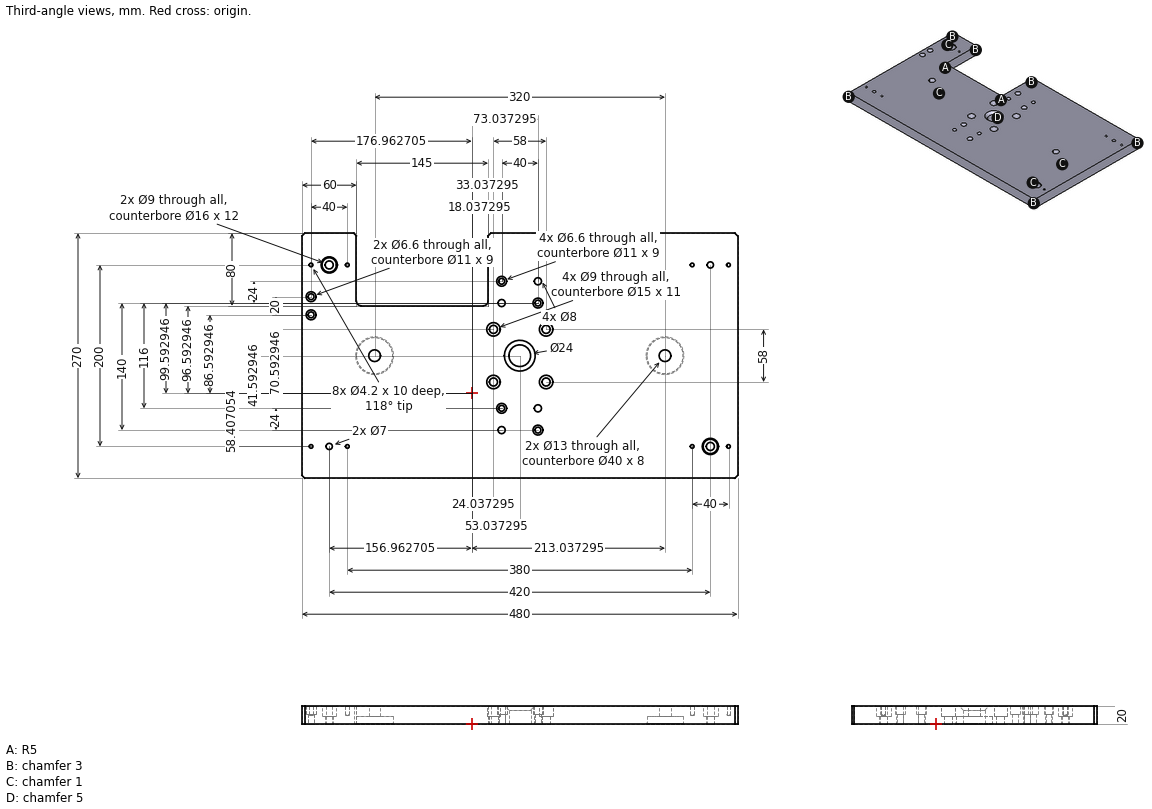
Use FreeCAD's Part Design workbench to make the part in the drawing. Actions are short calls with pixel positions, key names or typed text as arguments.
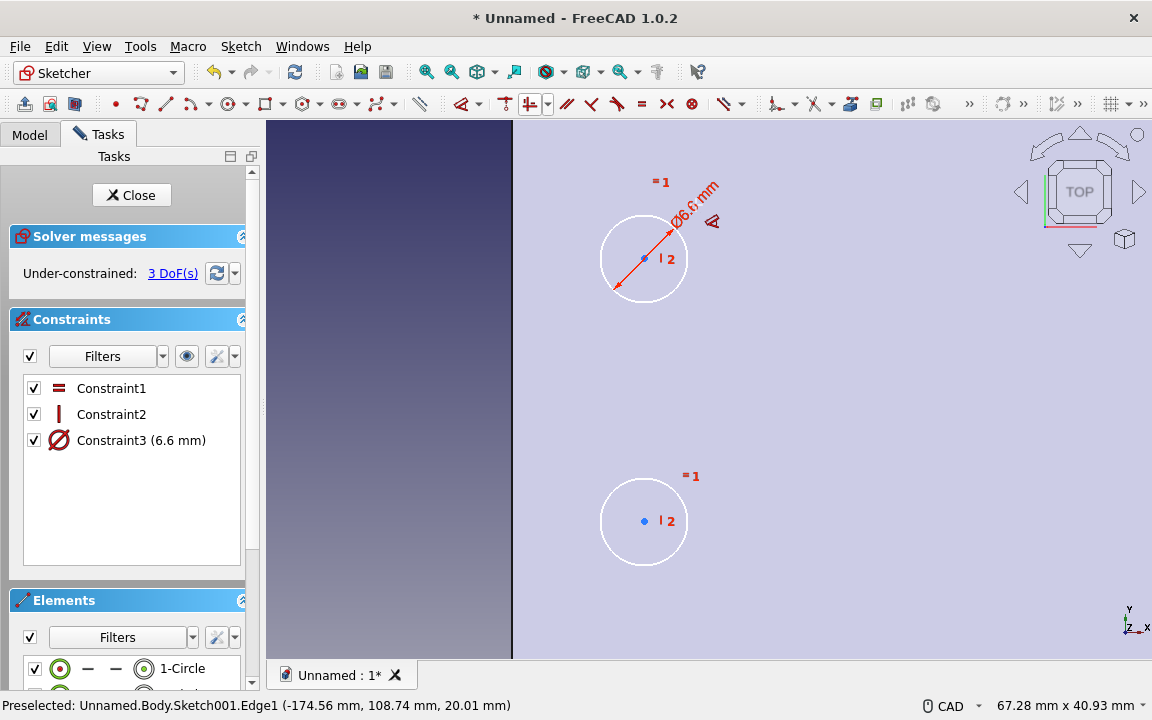
click(644, 259)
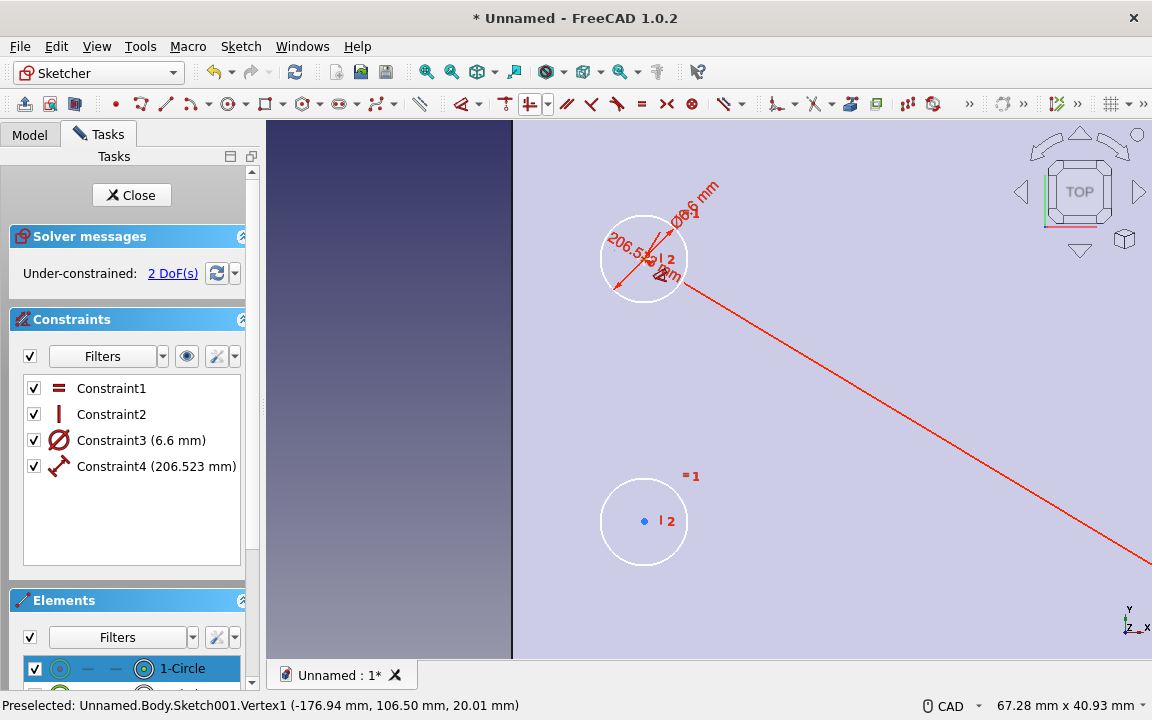
click(644, 522)
click(678, 390)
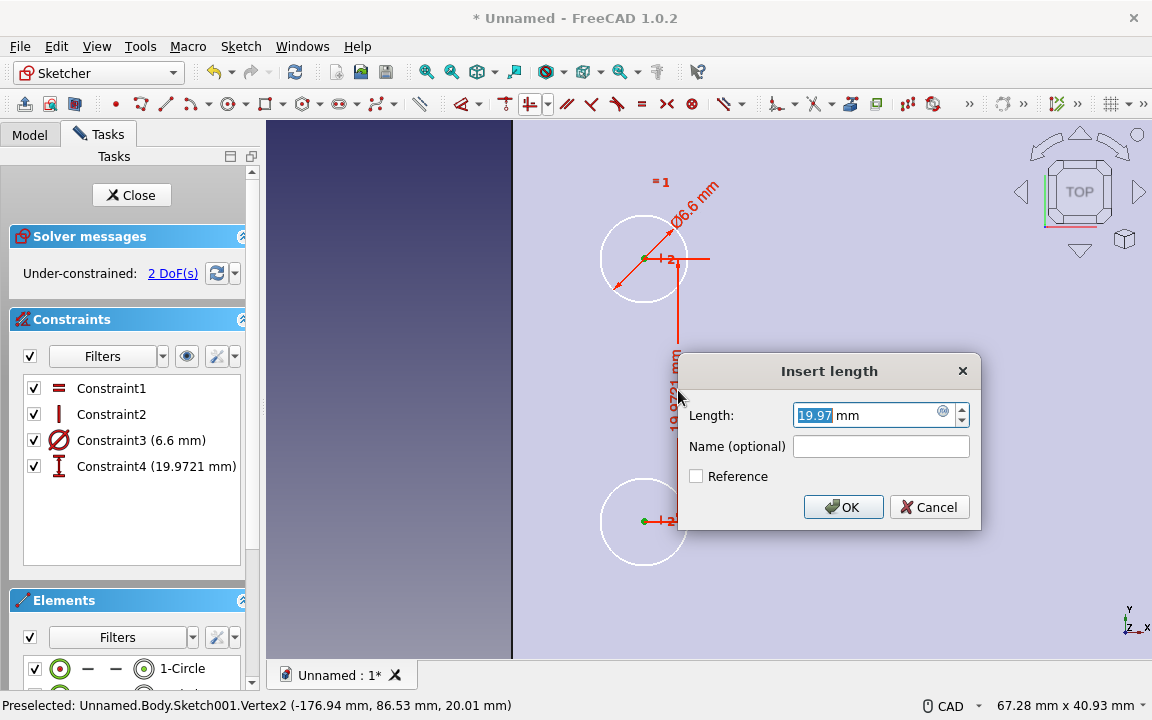
text(20)
key(Return)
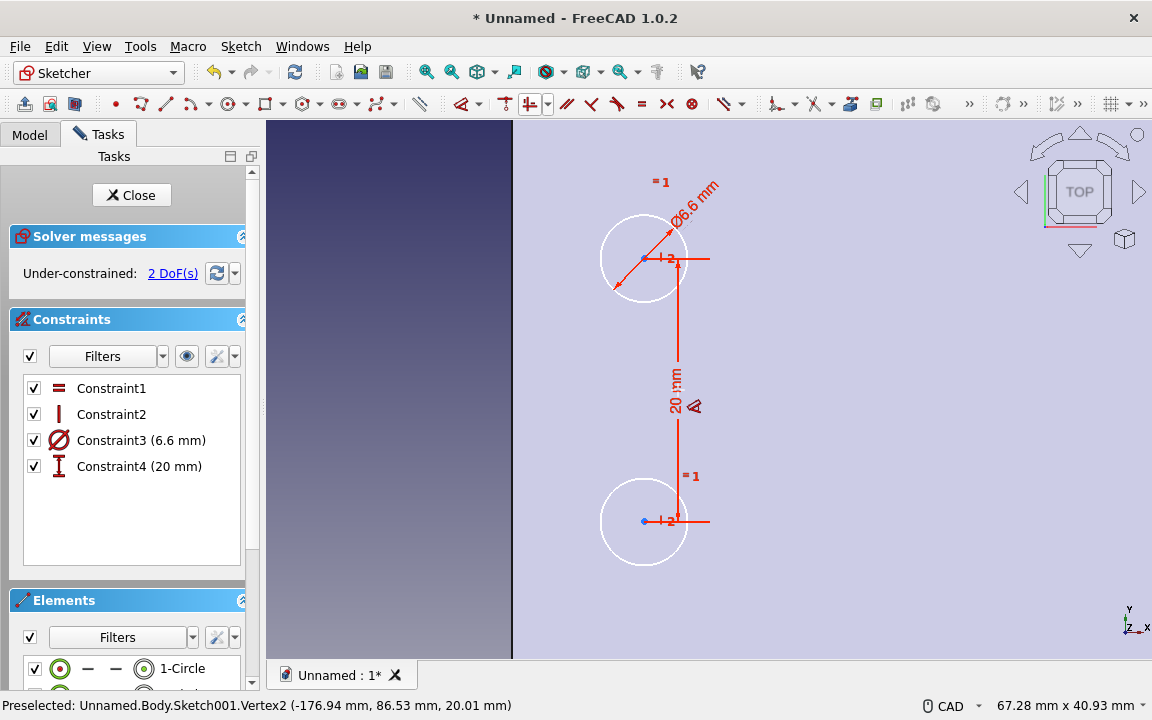
click(644, 522)
click(610, 576)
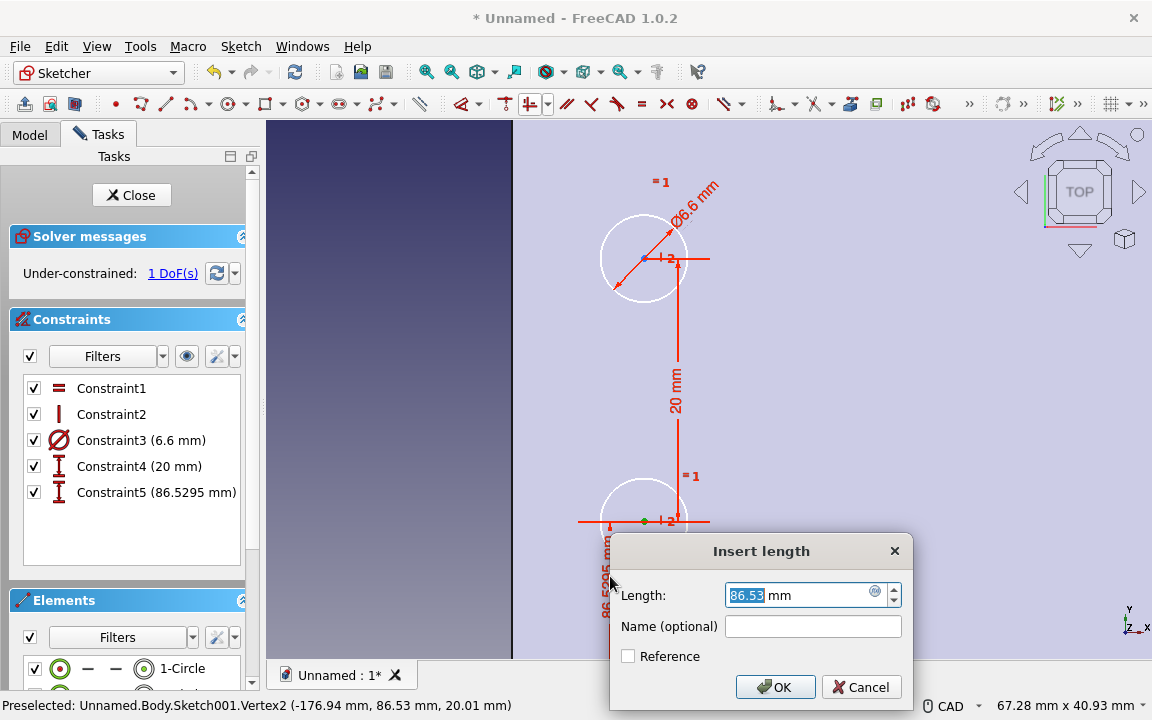
text(86.592946)
key(Return)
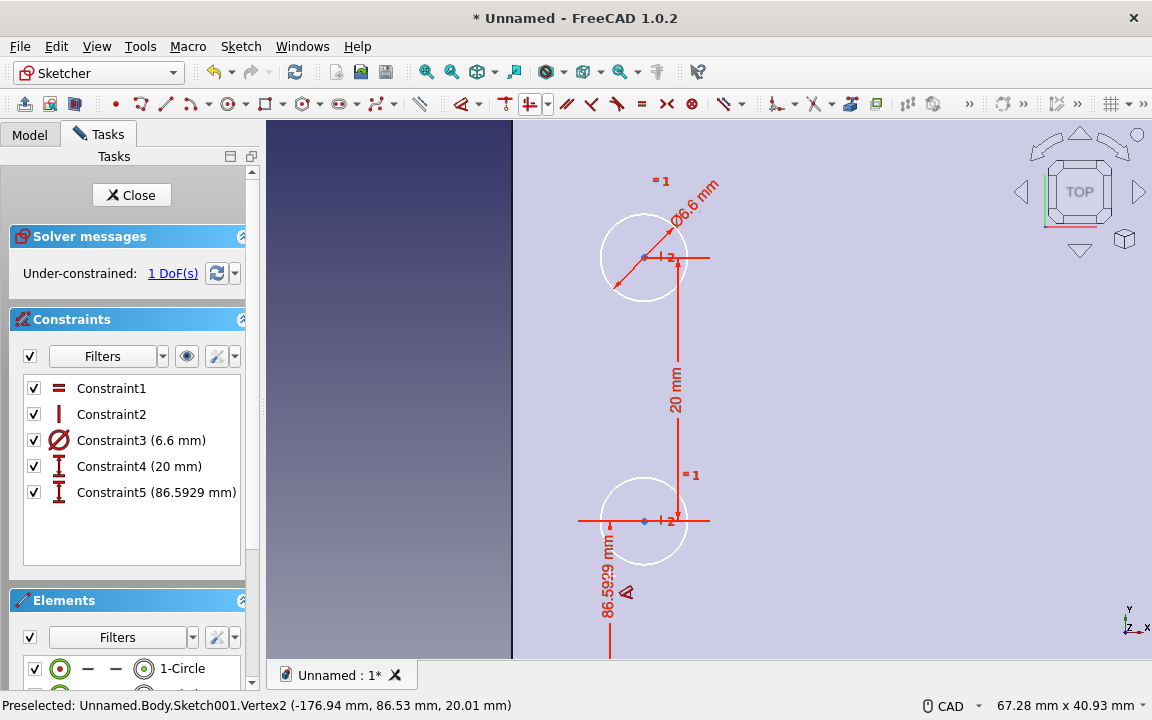
click(644, 258)
click(816, 224)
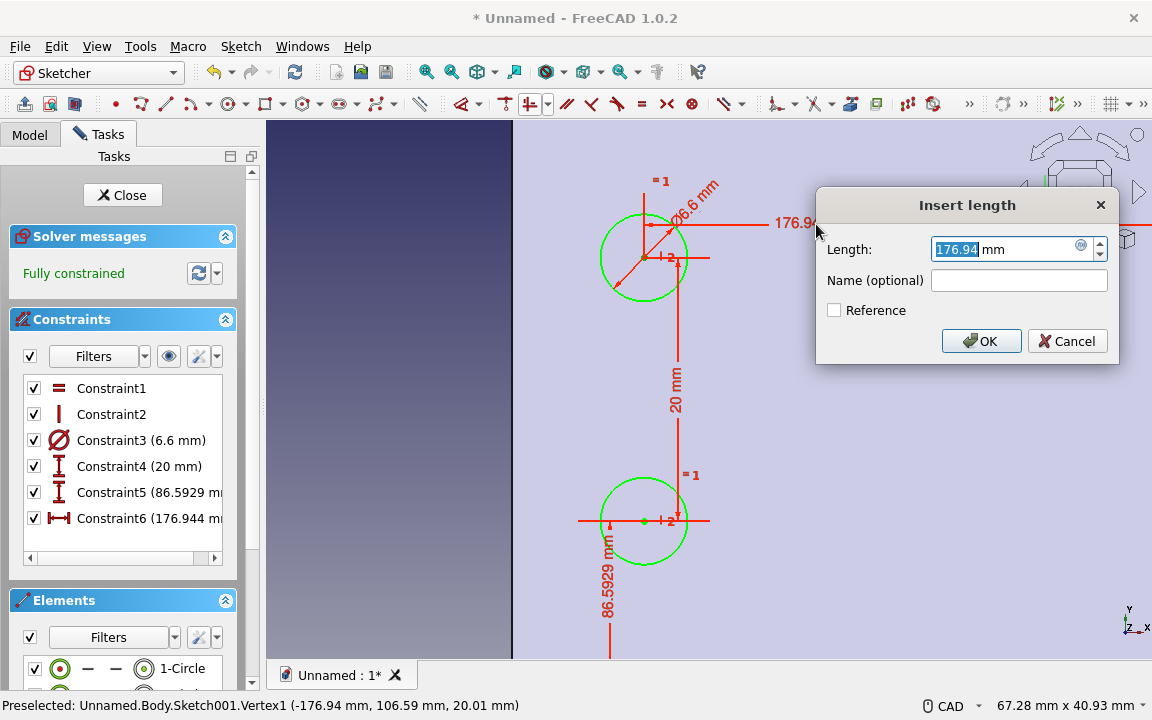
text(176.962705)
key(Return)
key(Escape)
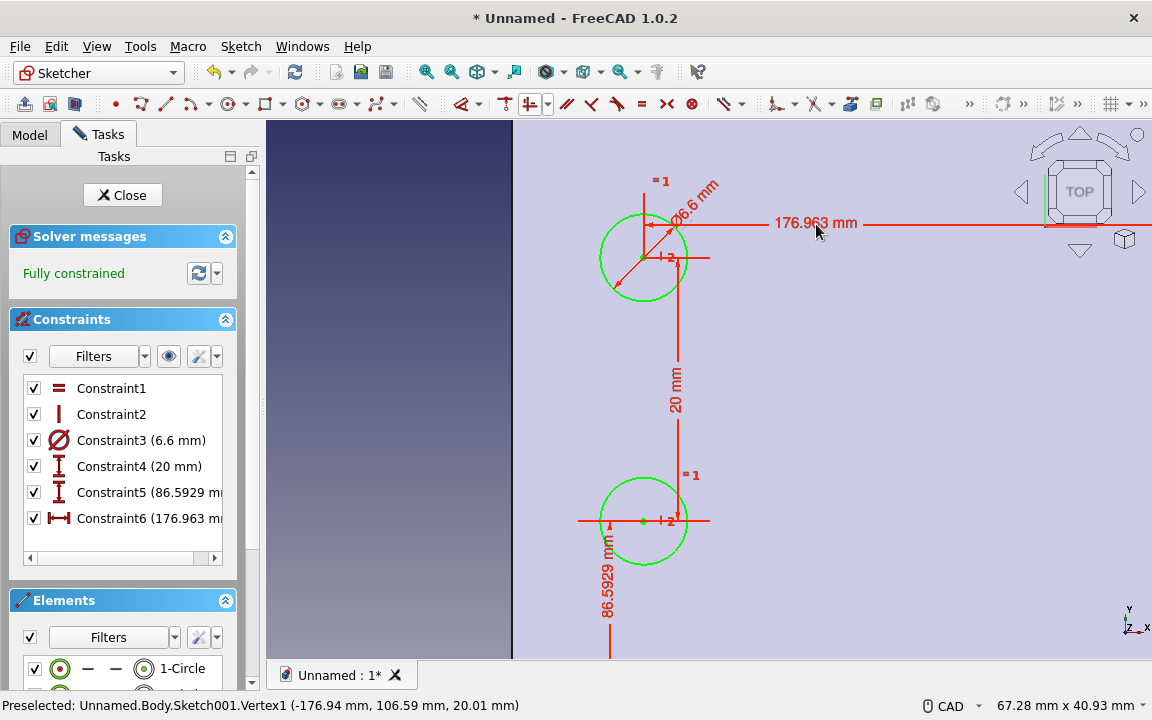
click(123, 195)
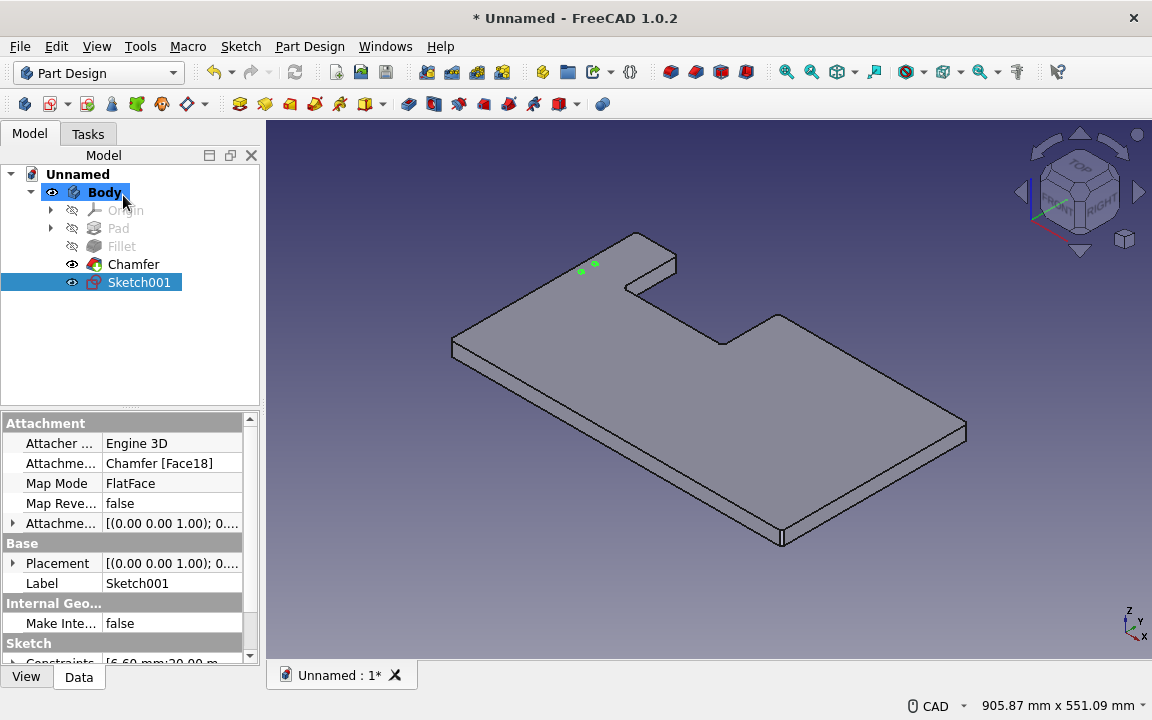
click(434, 104)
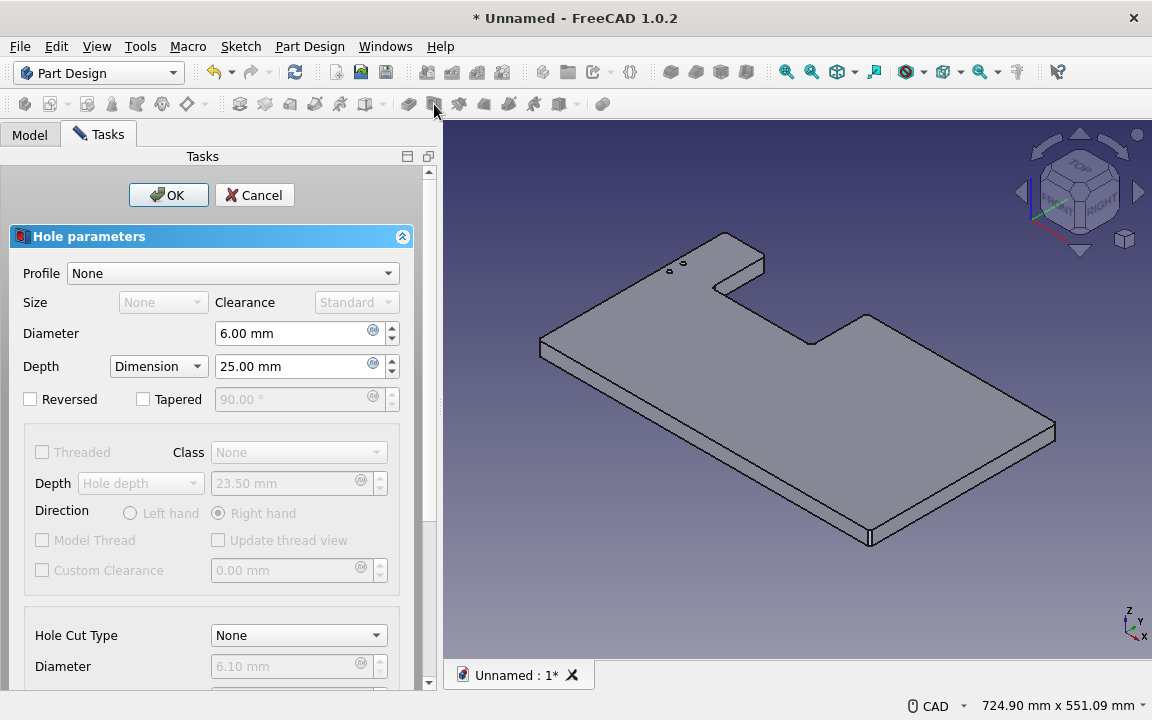
triple_click(300, 334)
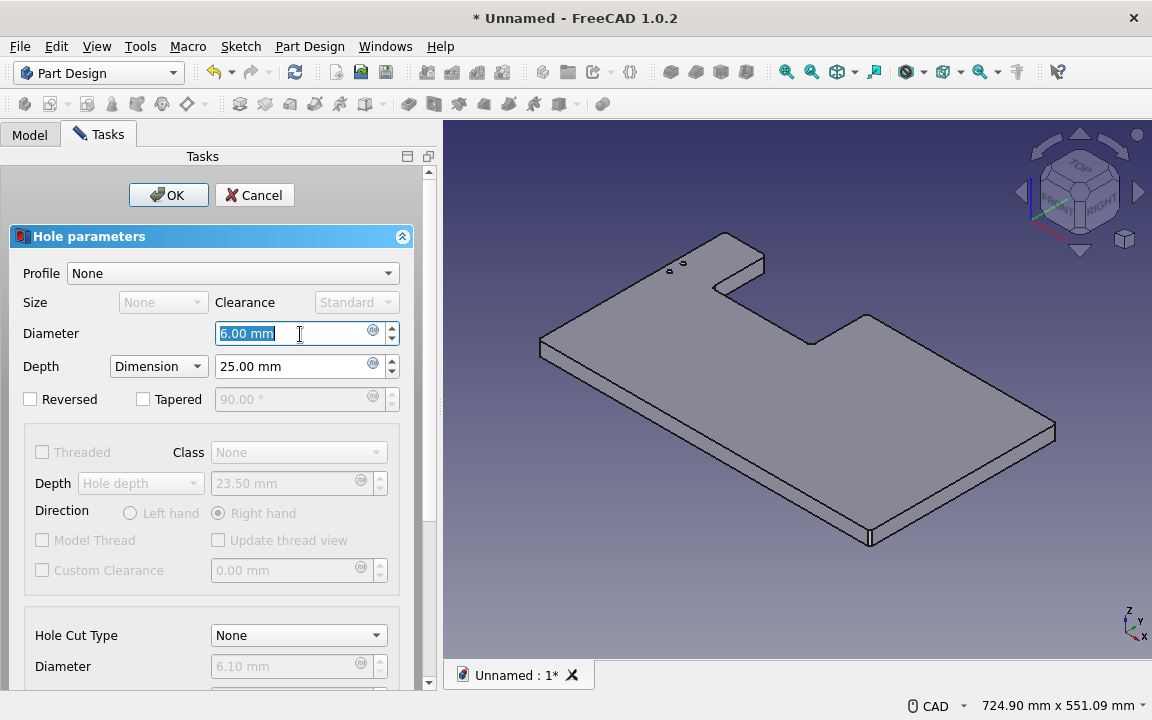
text(6.6)
key(Tab)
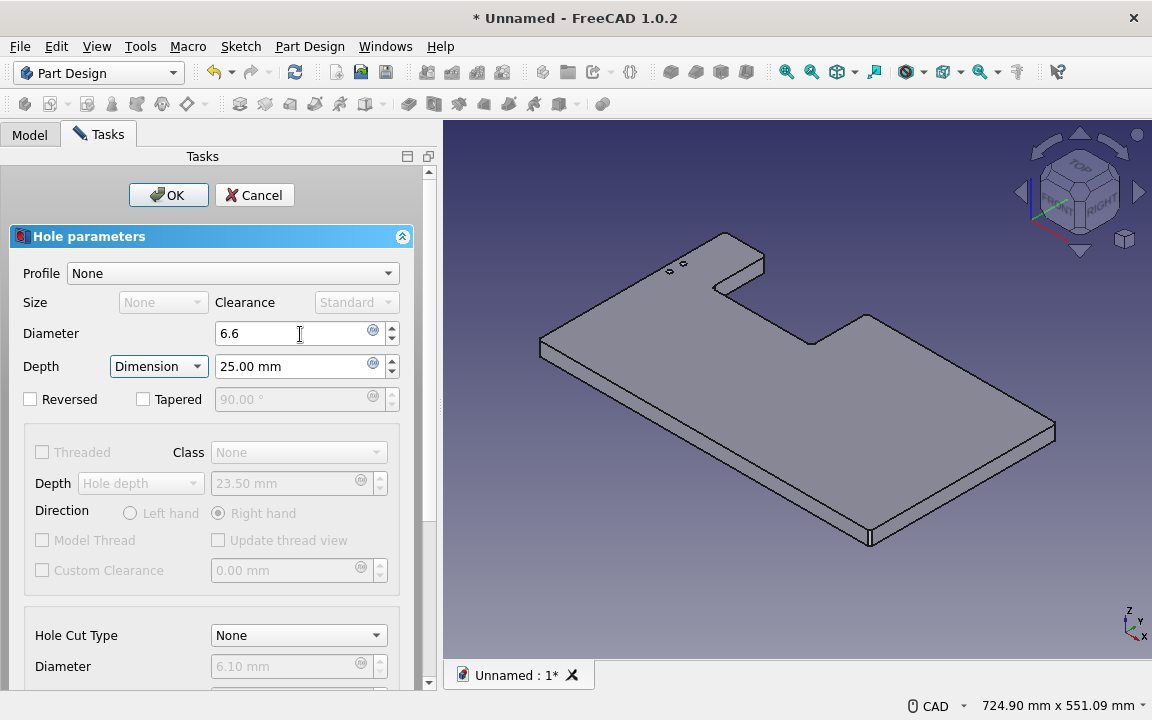
click(160, 366)